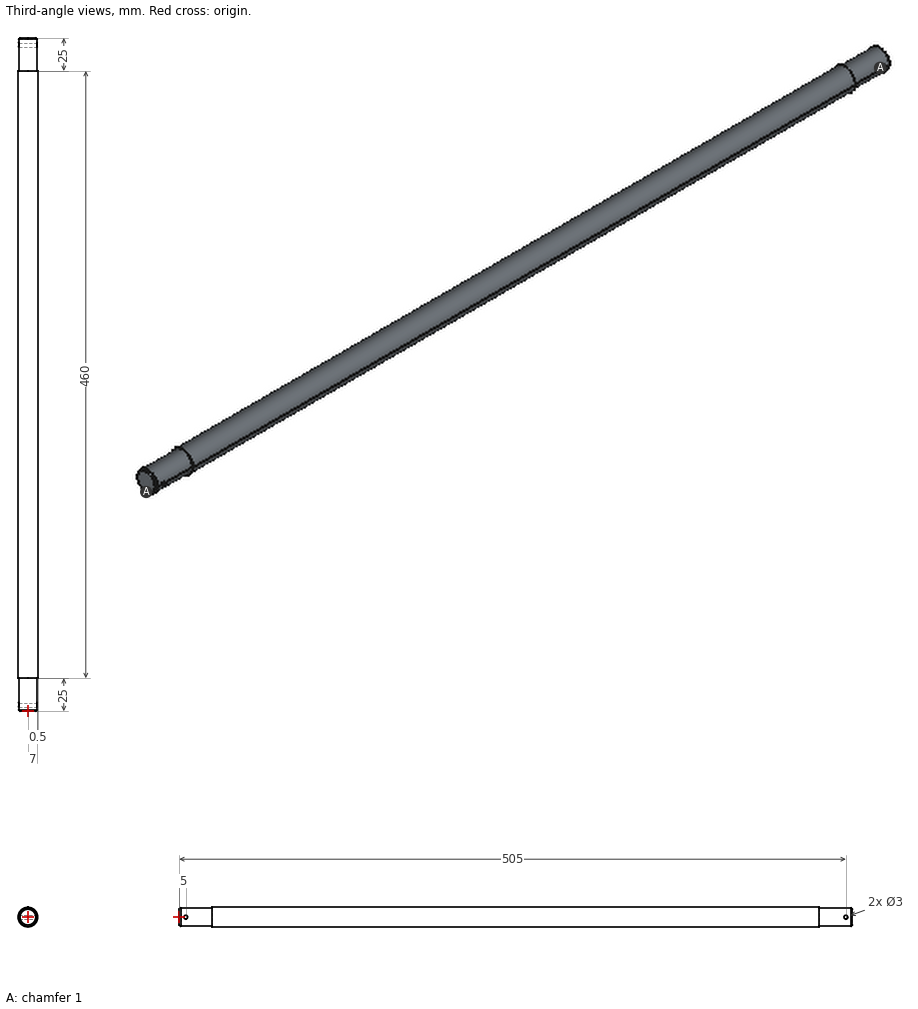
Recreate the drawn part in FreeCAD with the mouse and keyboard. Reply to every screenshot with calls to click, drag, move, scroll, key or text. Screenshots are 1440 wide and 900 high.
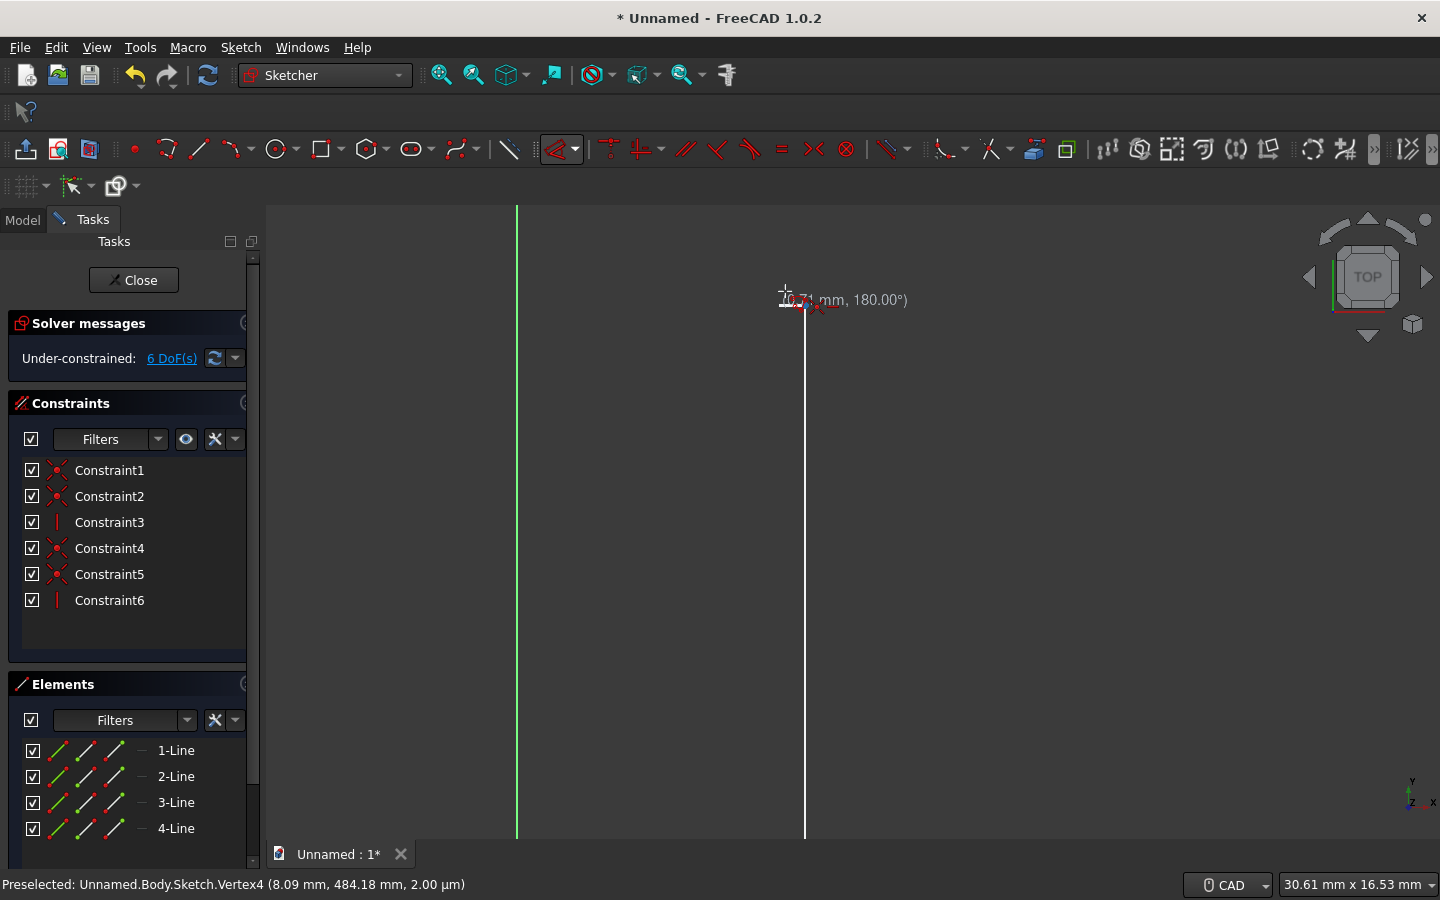
click(786, 289)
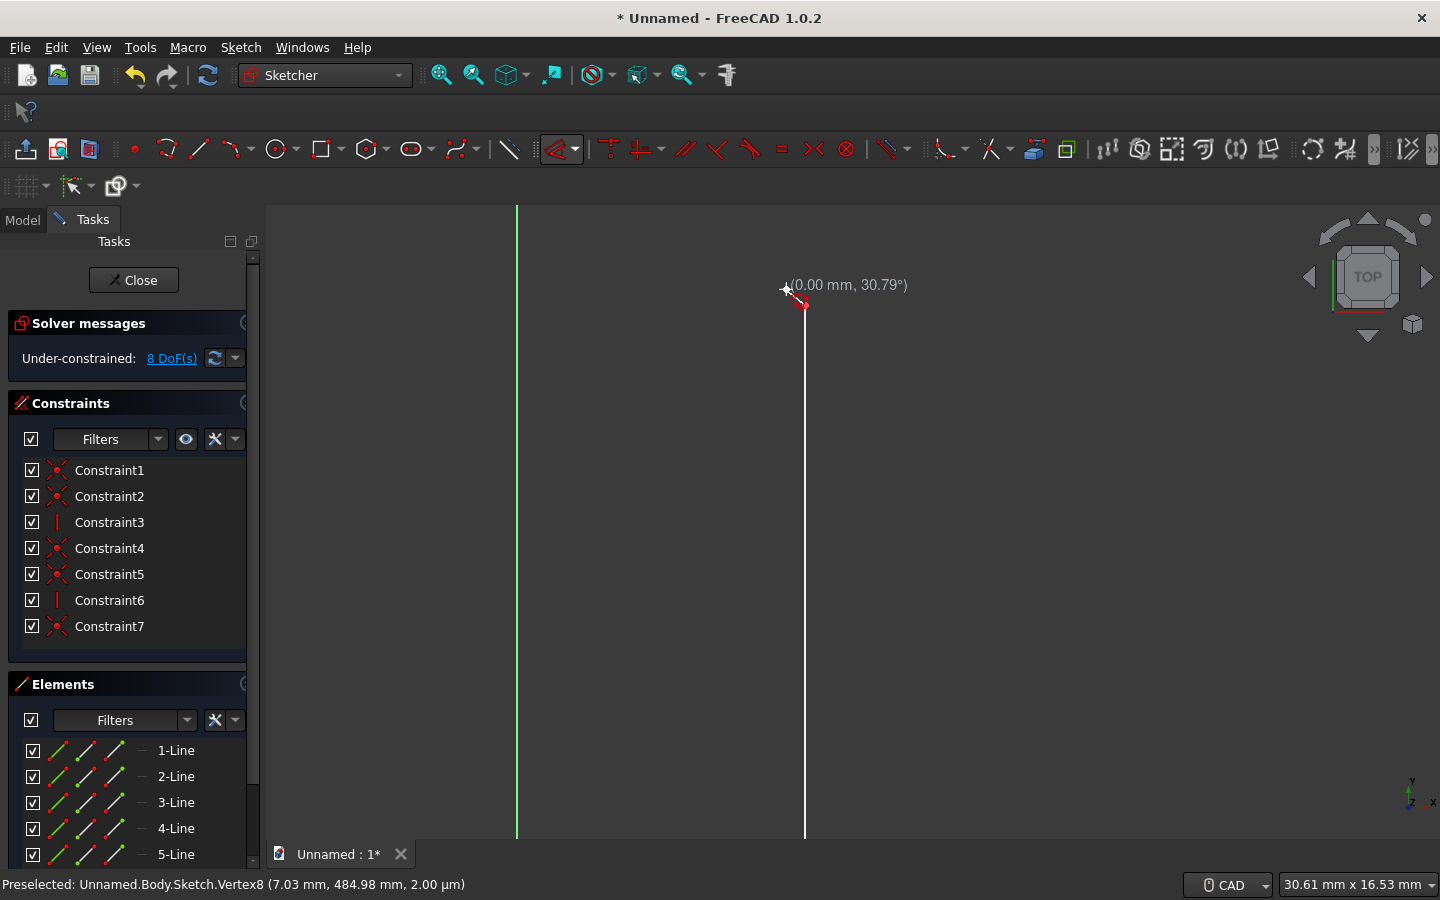
scroll(784, 522, down, 15)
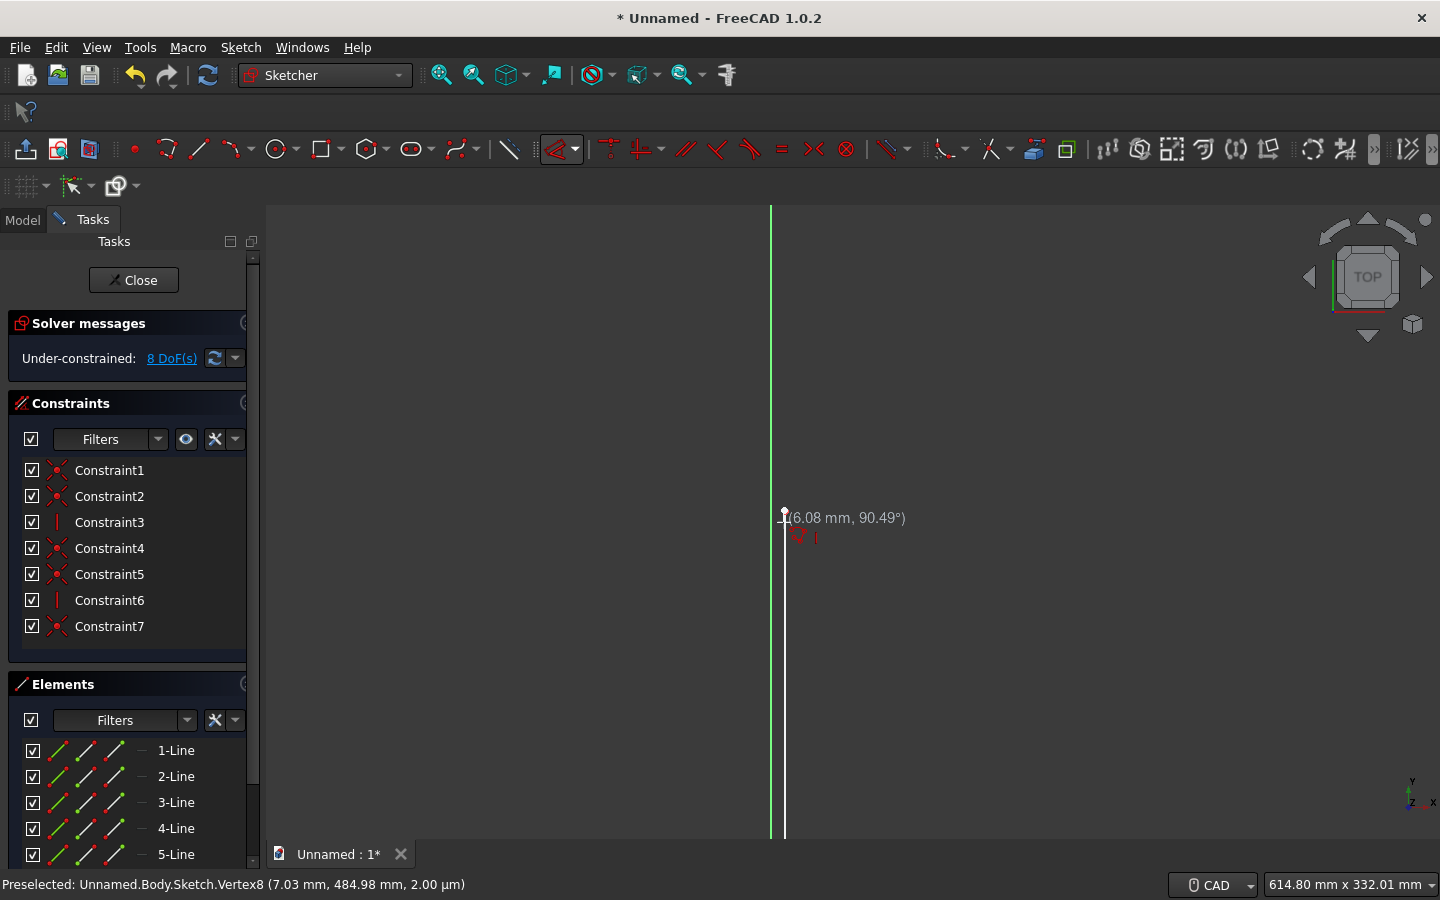
scroll(790, 233, down, 4)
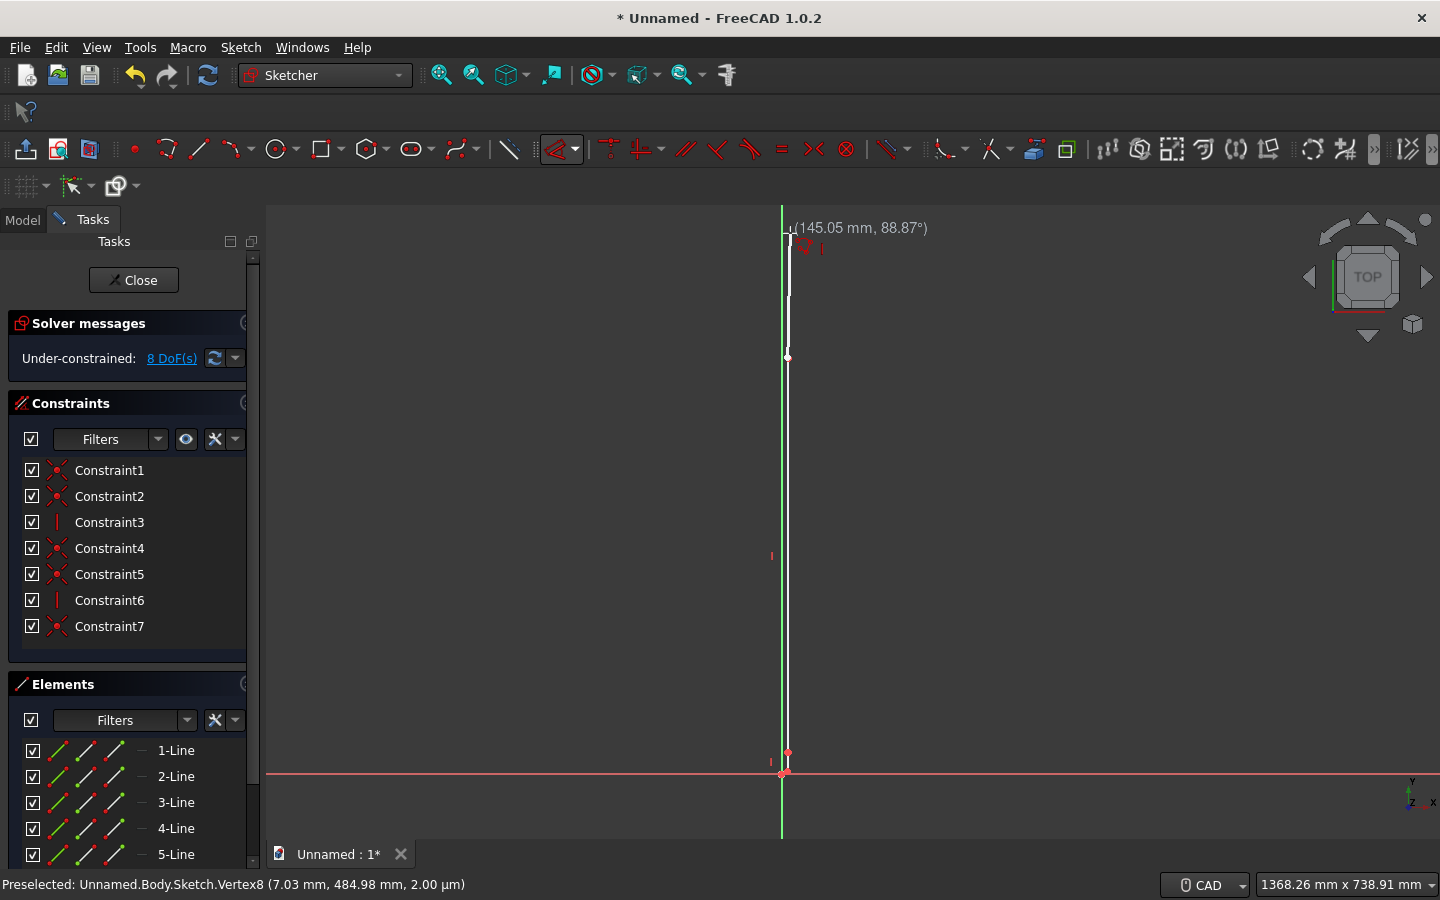
scroll(788, 336, up, 5)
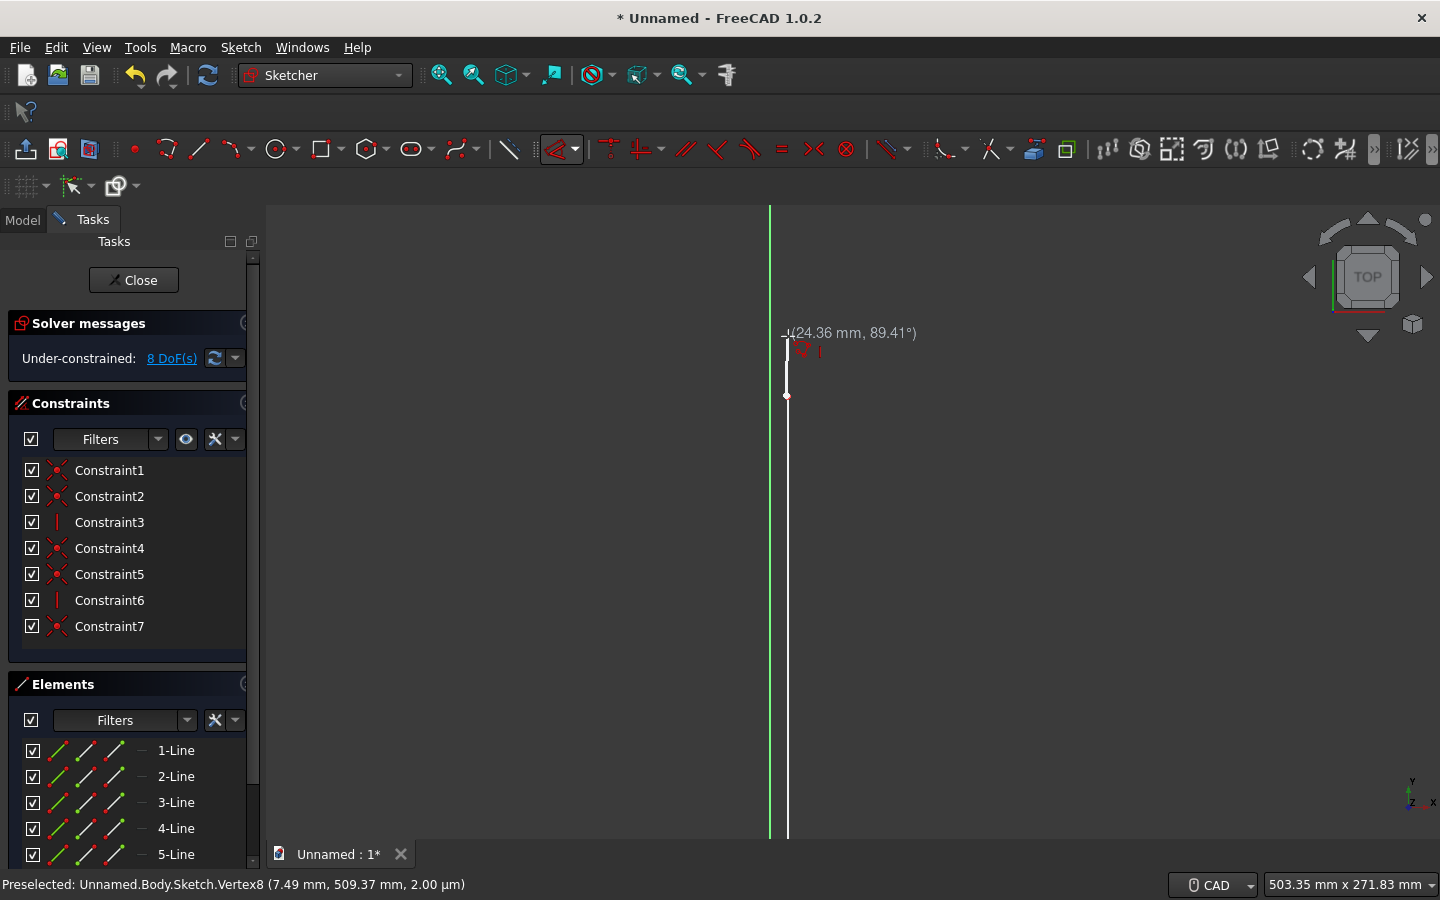
click(787, 337)
click(779, 337)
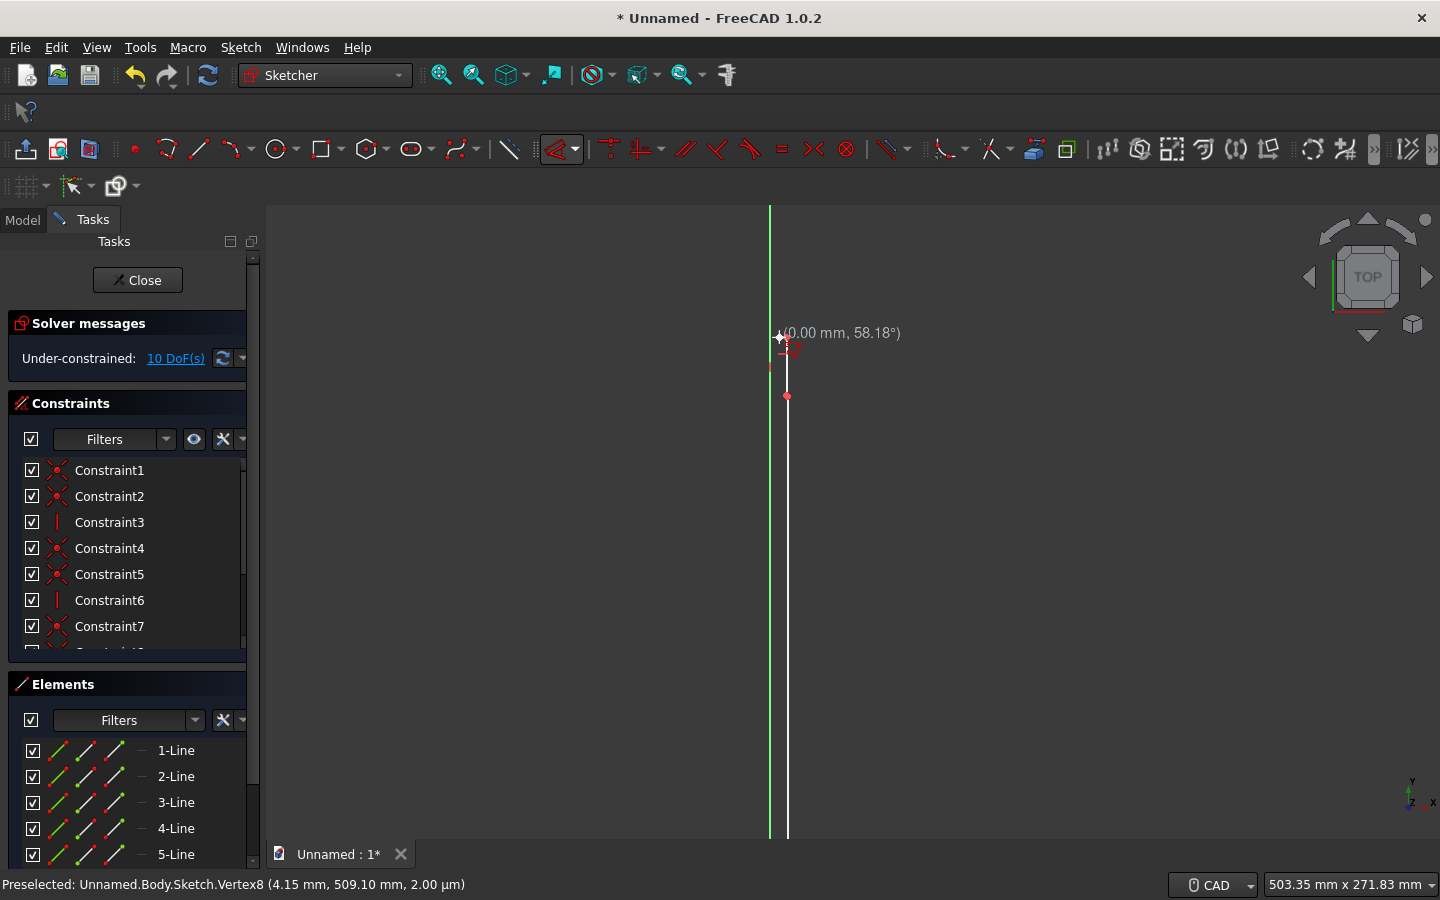
scroll(788, 284, down, 5)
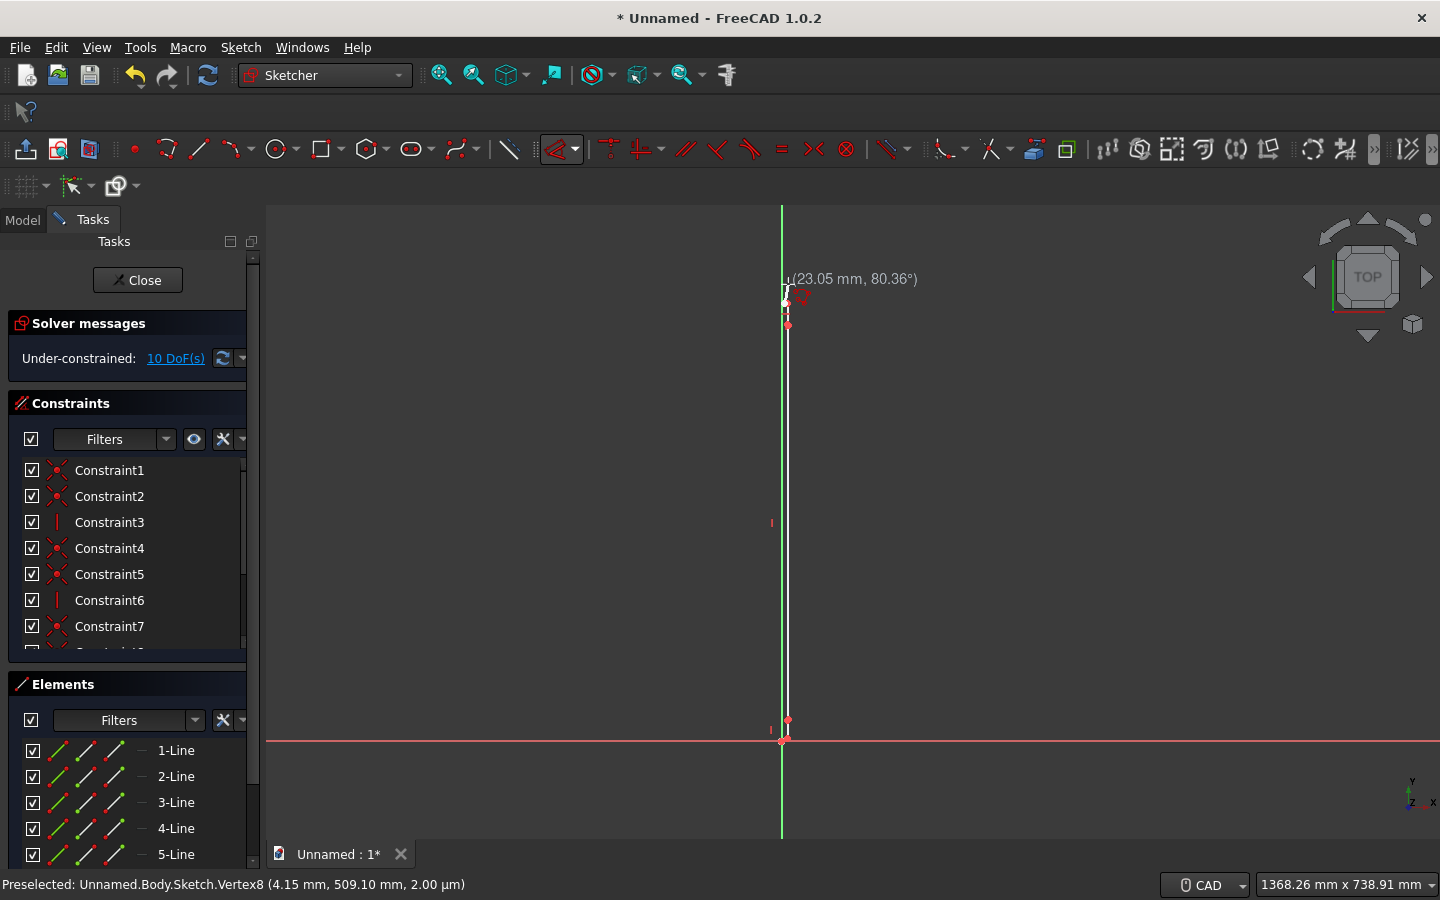
scroll(782, 741, up, 9)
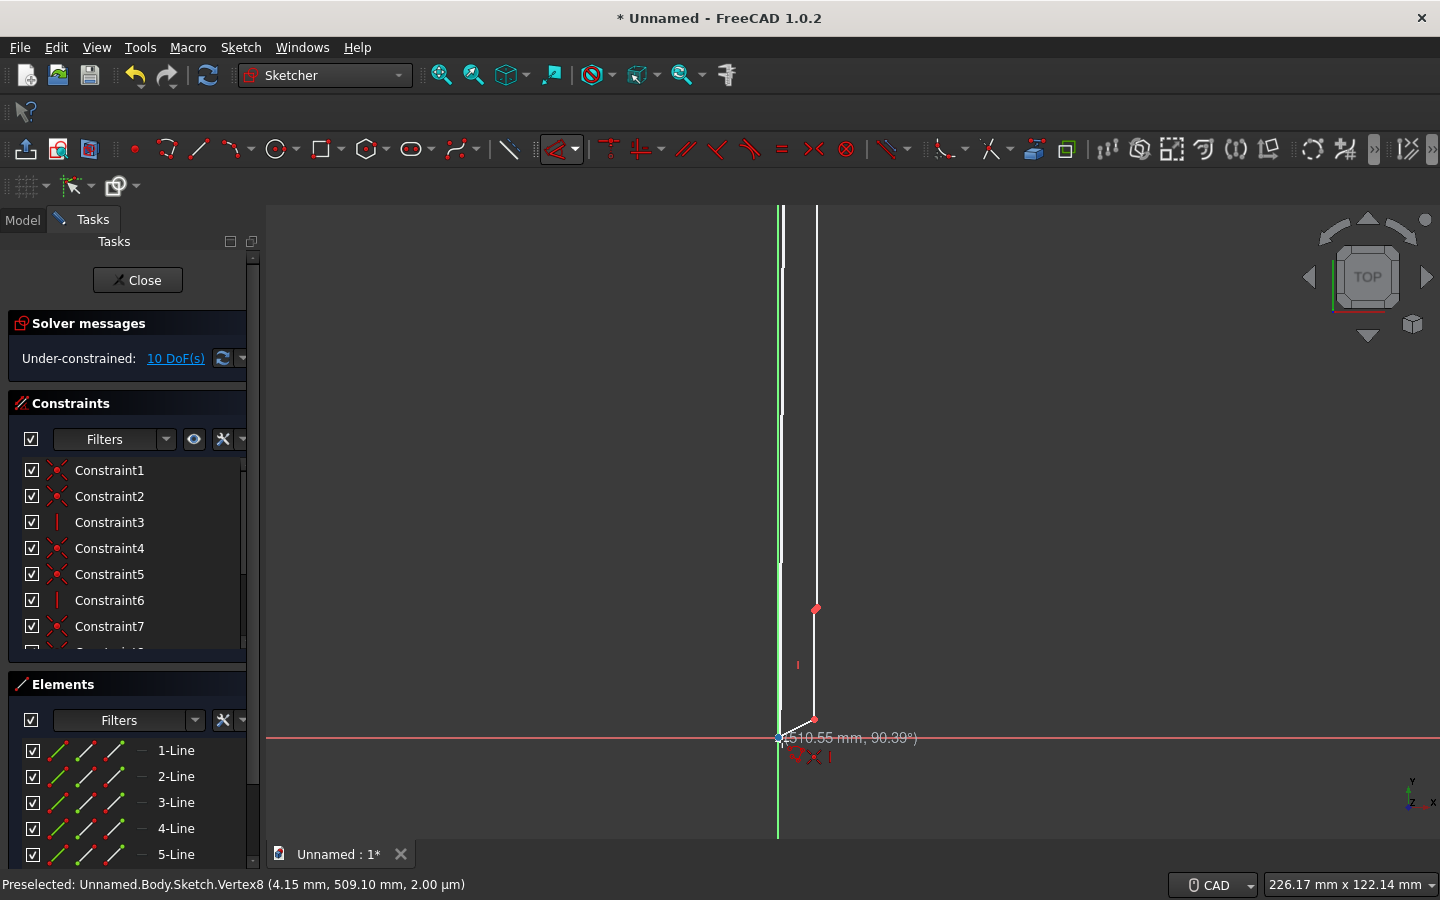
click(778, 738)
key(Escape)
key(Escape)